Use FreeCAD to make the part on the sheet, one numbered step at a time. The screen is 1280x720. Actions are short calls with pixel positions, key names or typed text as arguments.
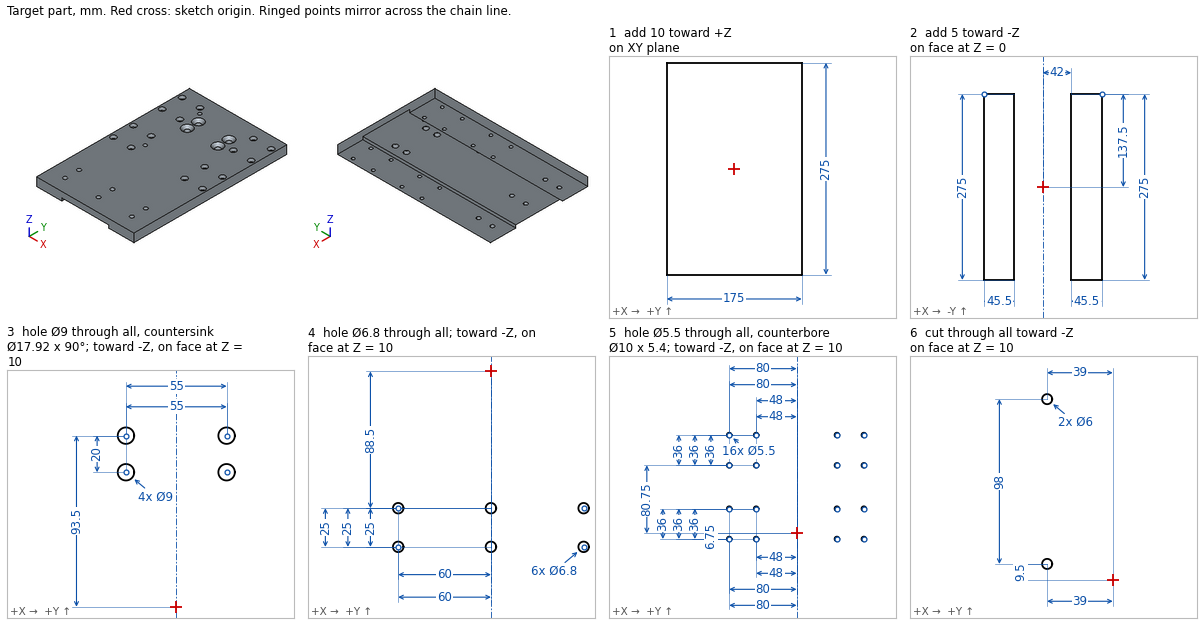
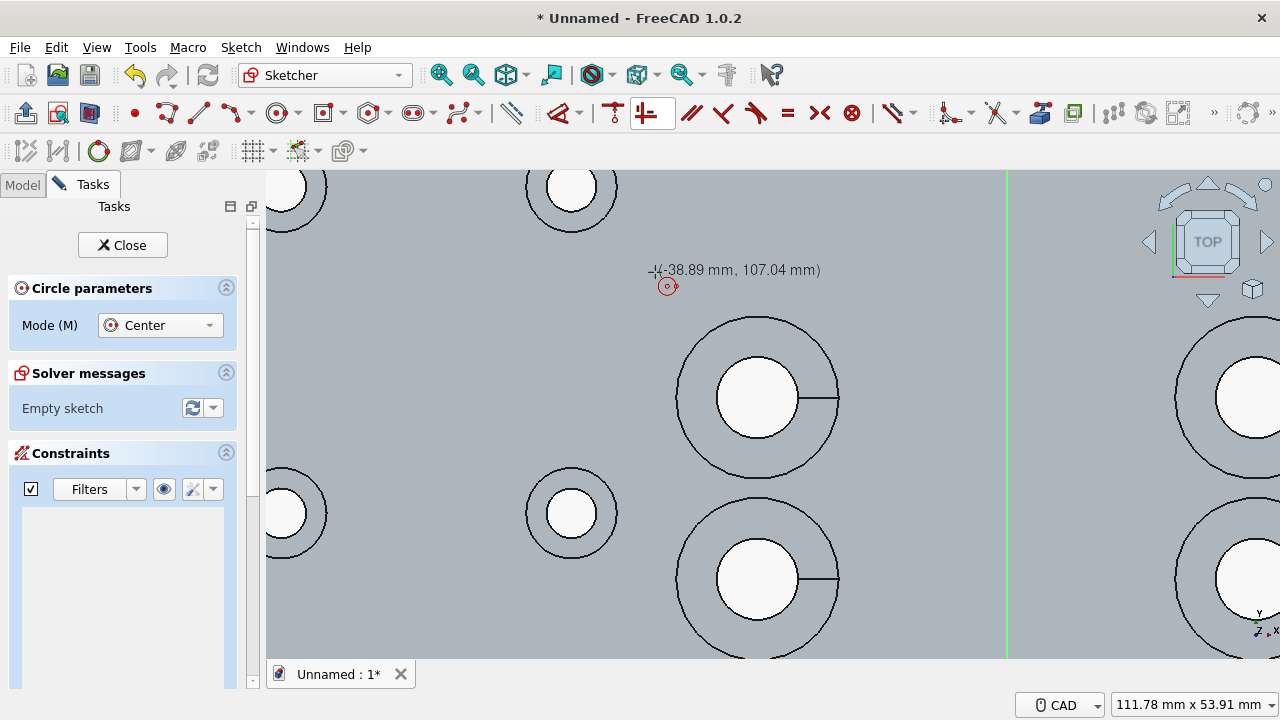
click(653, 271)
move(672, 251)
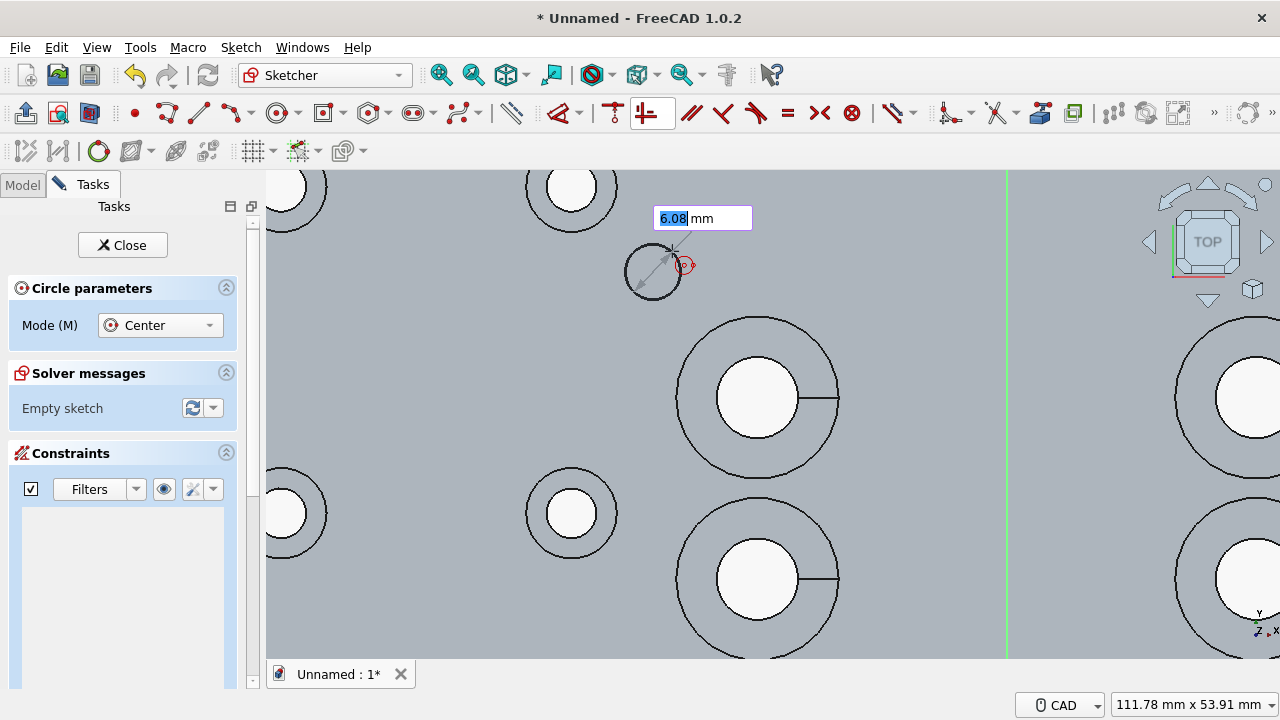
text(6)
key(Return)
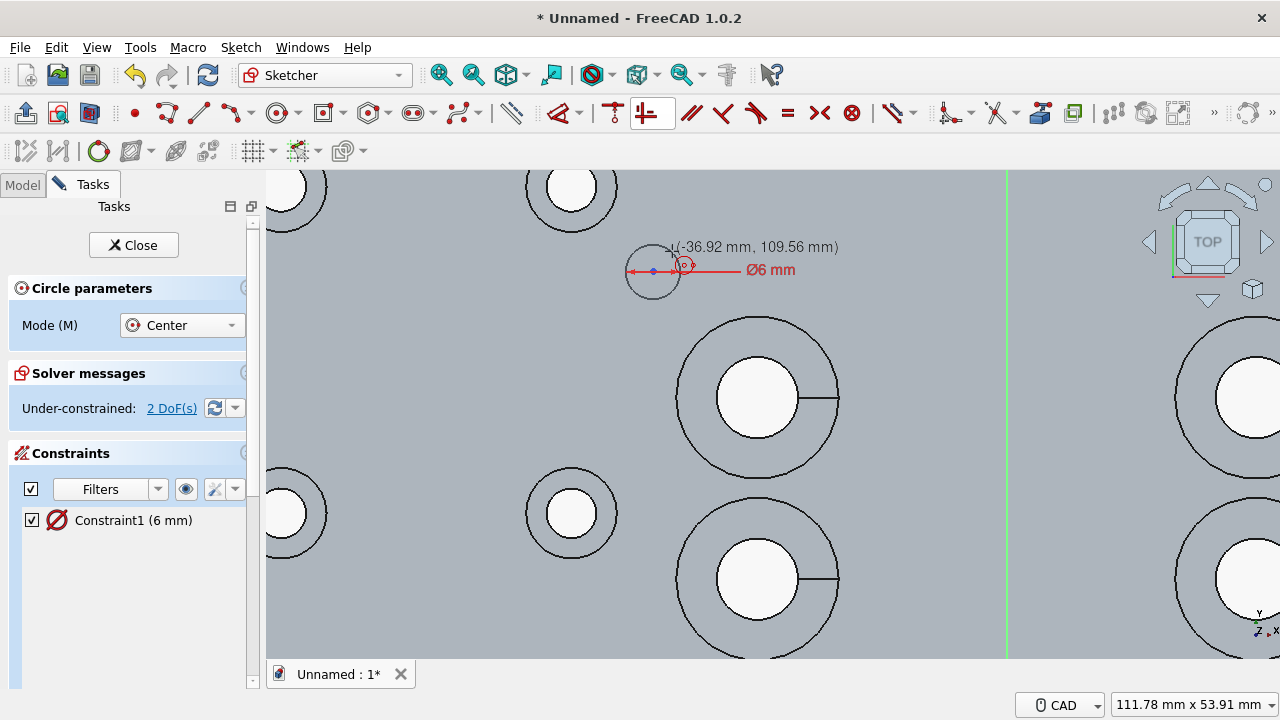
scroll(656, 272, down, 6)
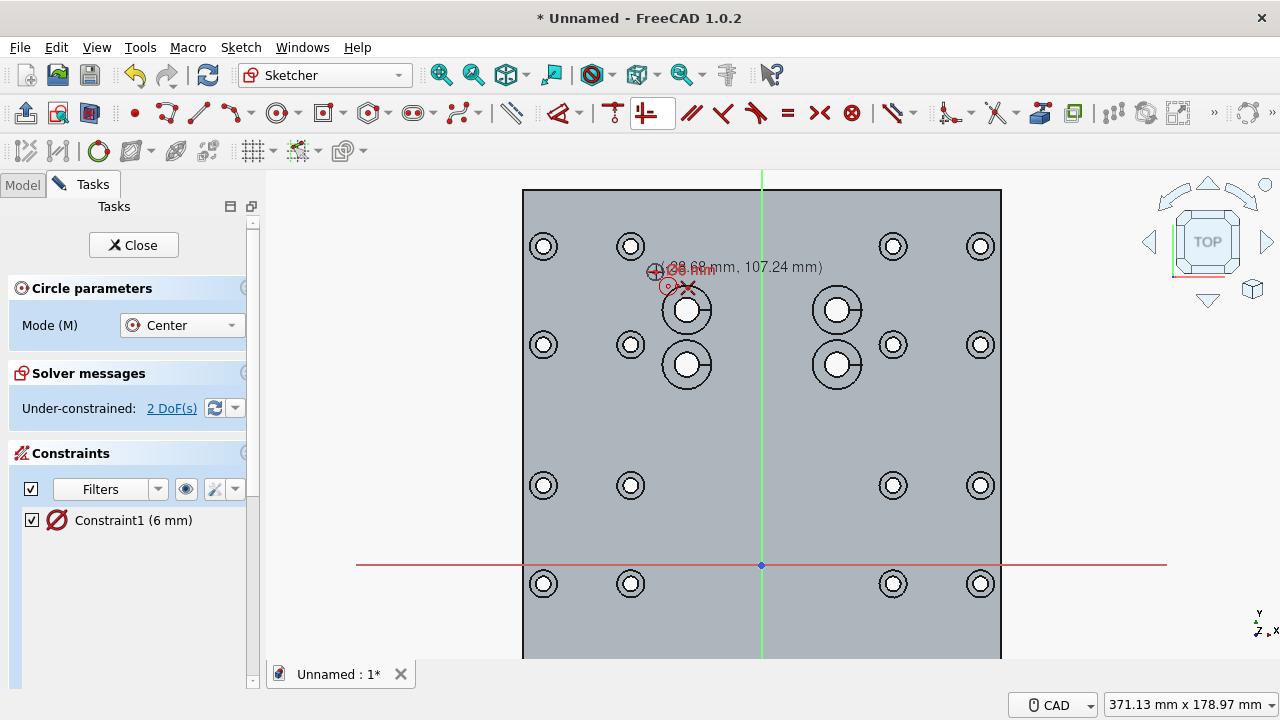
scroll(655, 539, up, 6)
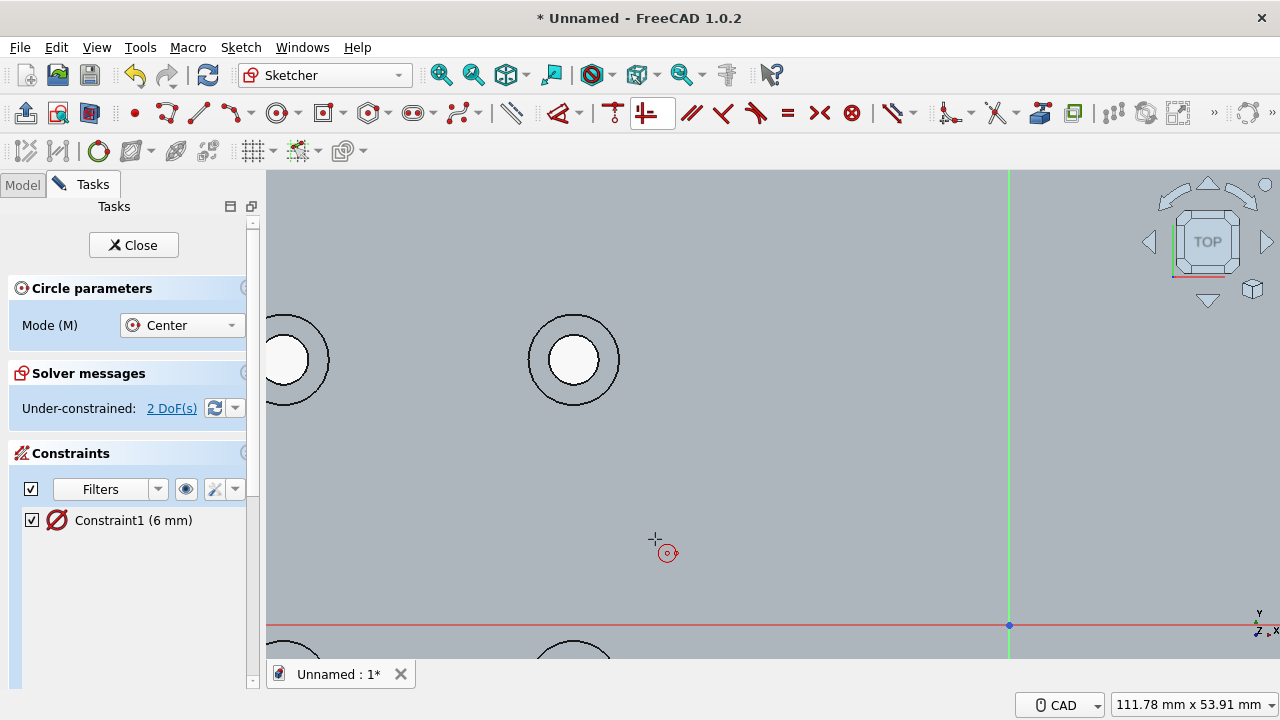
click(655, 539)
move(675, 520)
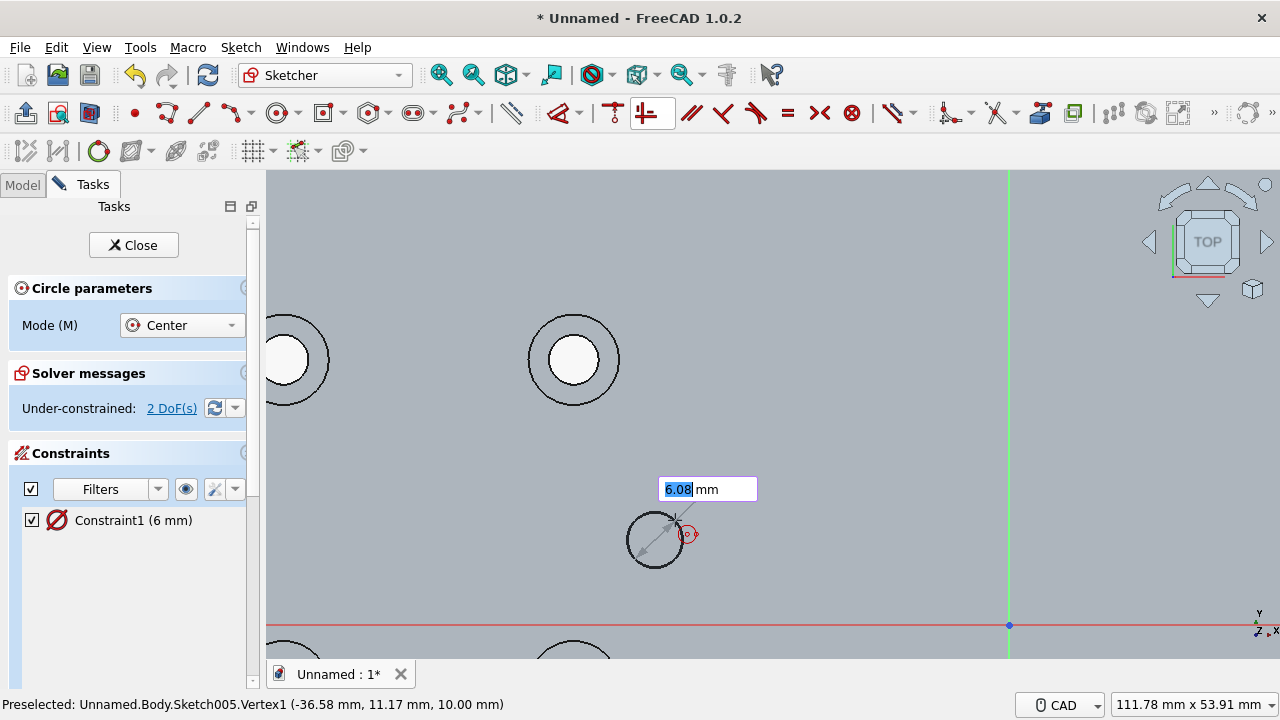
text(6)
key(Return)
key(Escape)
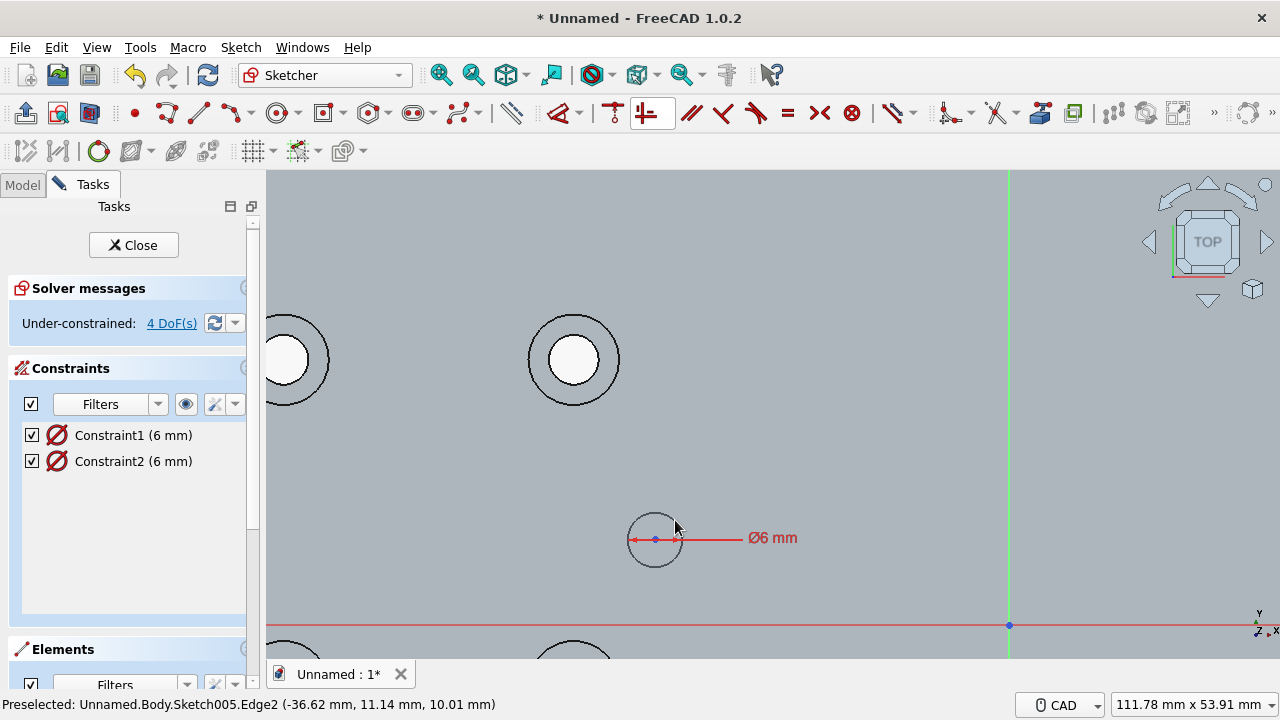
key(d)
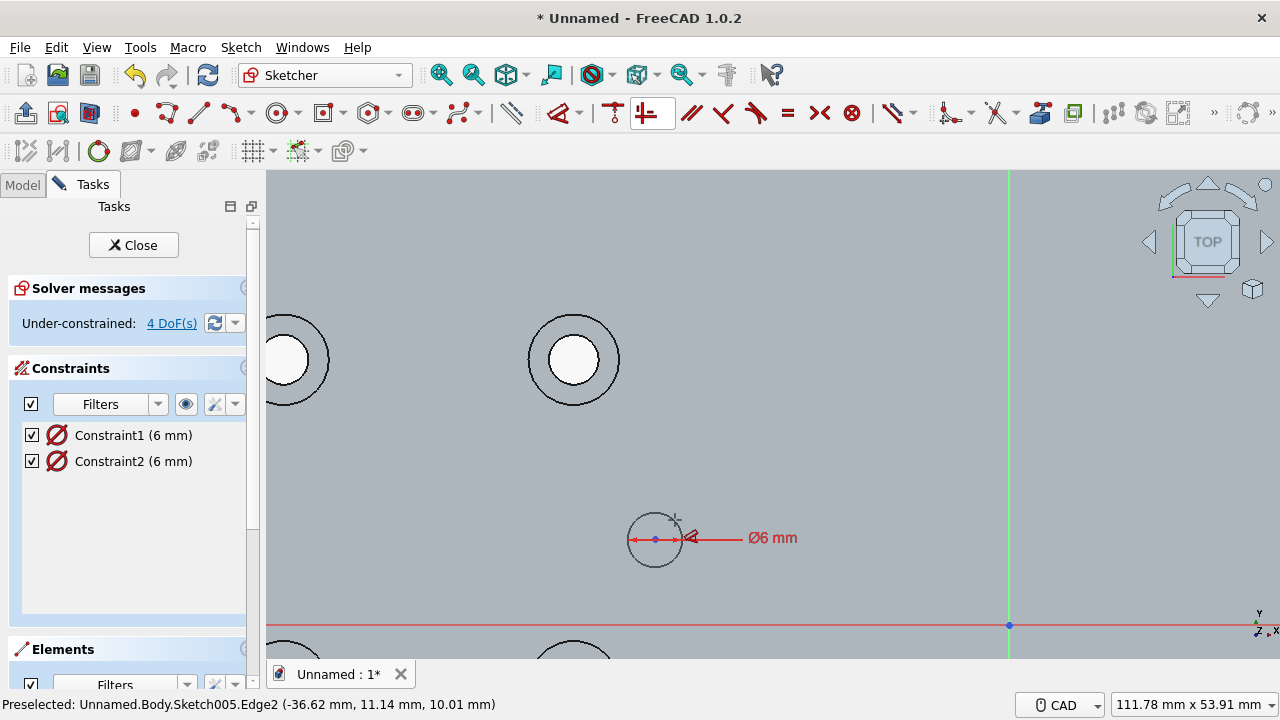
scroll(655, 540, down, 6)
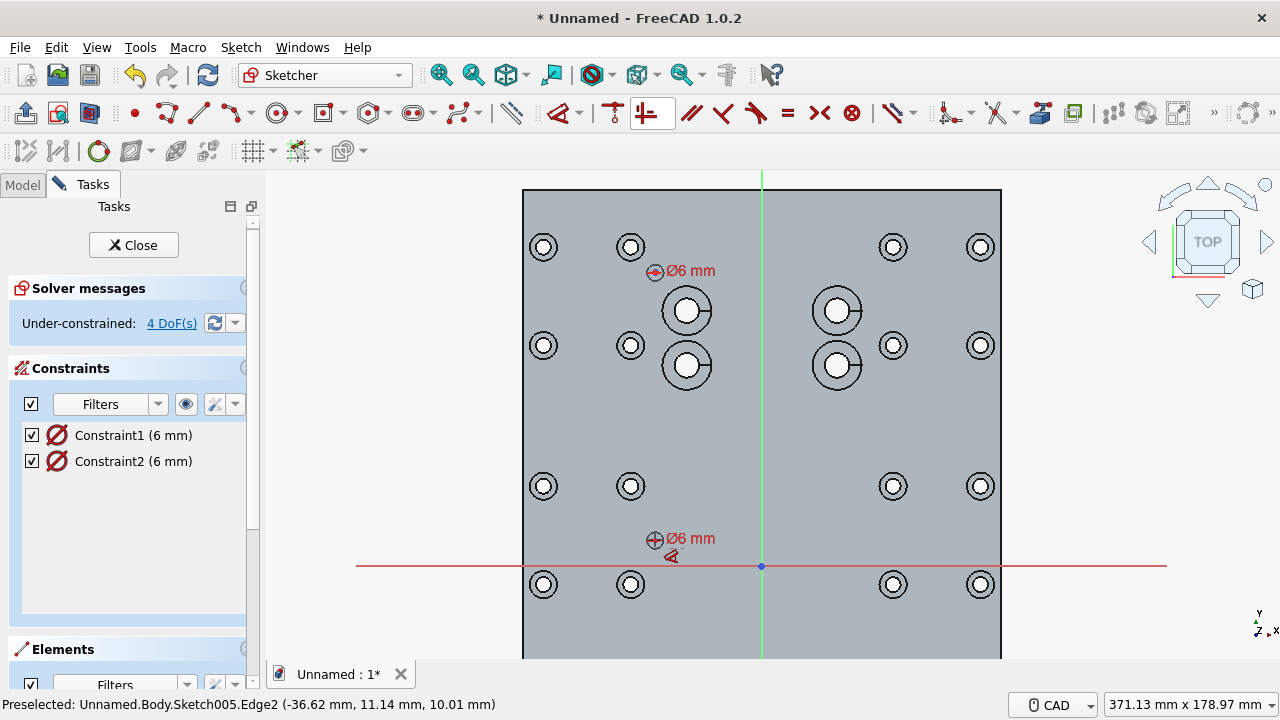
click(655, 273)
click(709, 600)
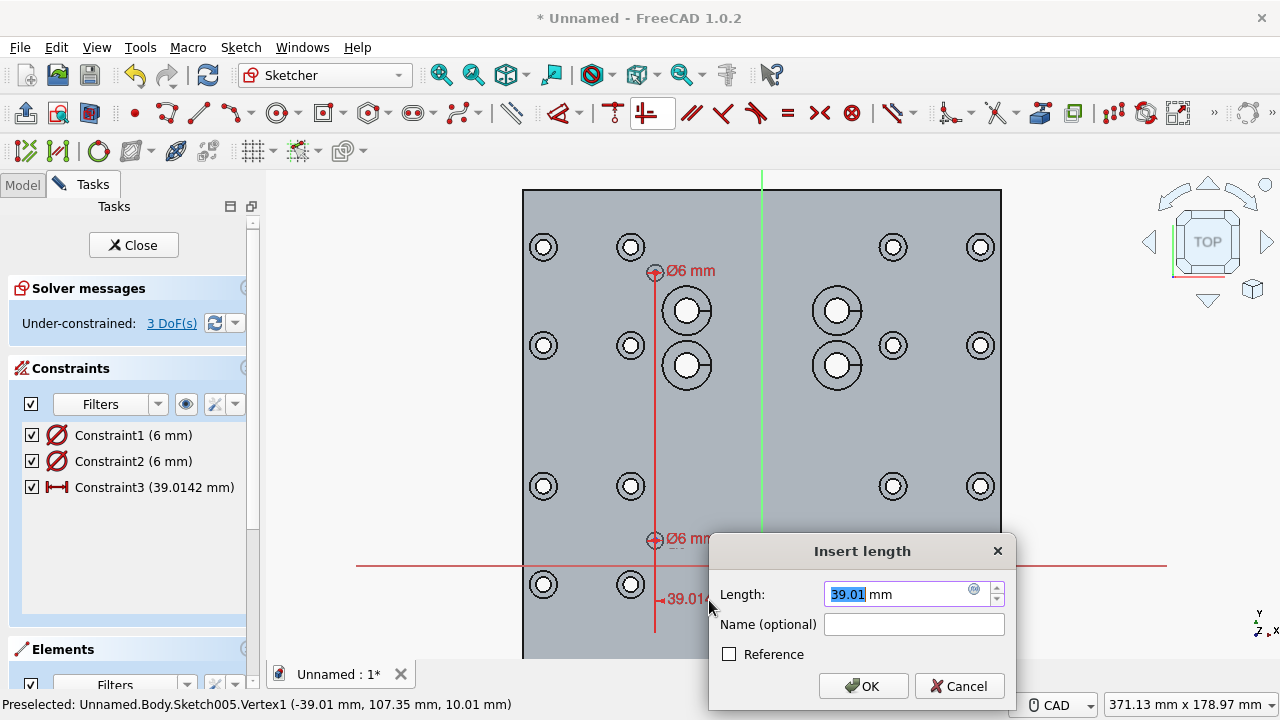
text(39)
key(Return)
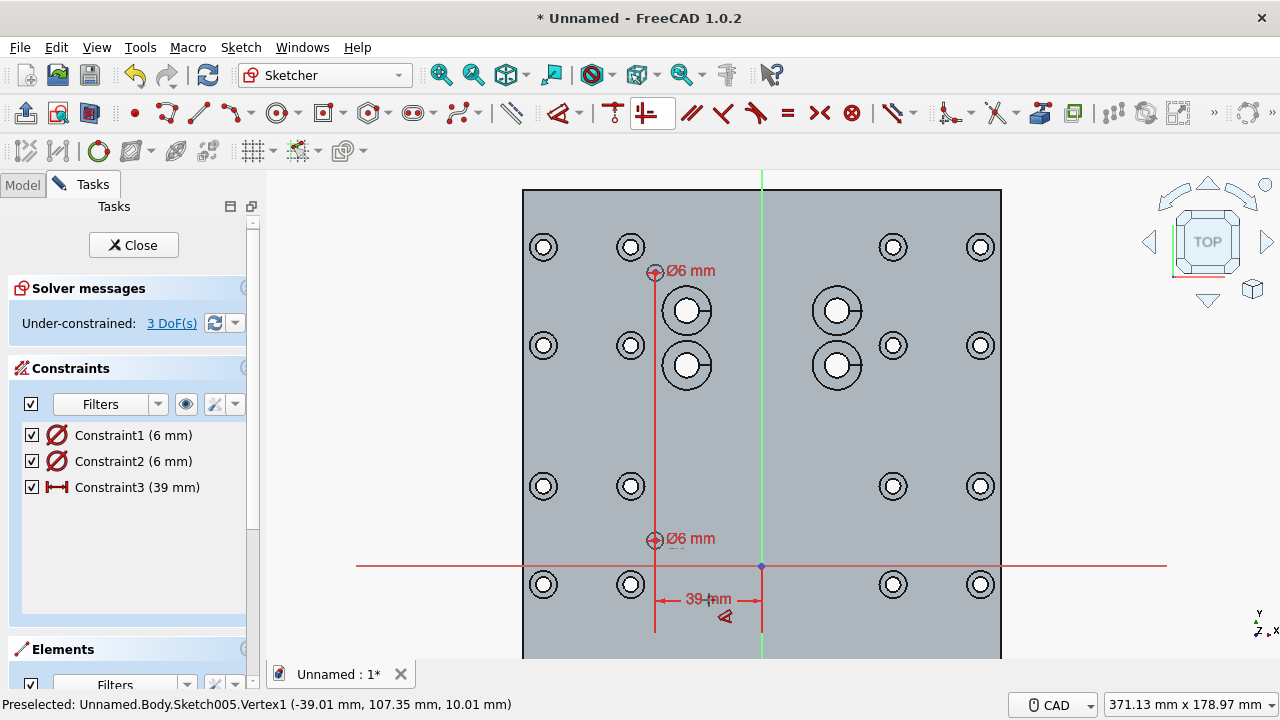
click(655, 541)
click(709, 507)